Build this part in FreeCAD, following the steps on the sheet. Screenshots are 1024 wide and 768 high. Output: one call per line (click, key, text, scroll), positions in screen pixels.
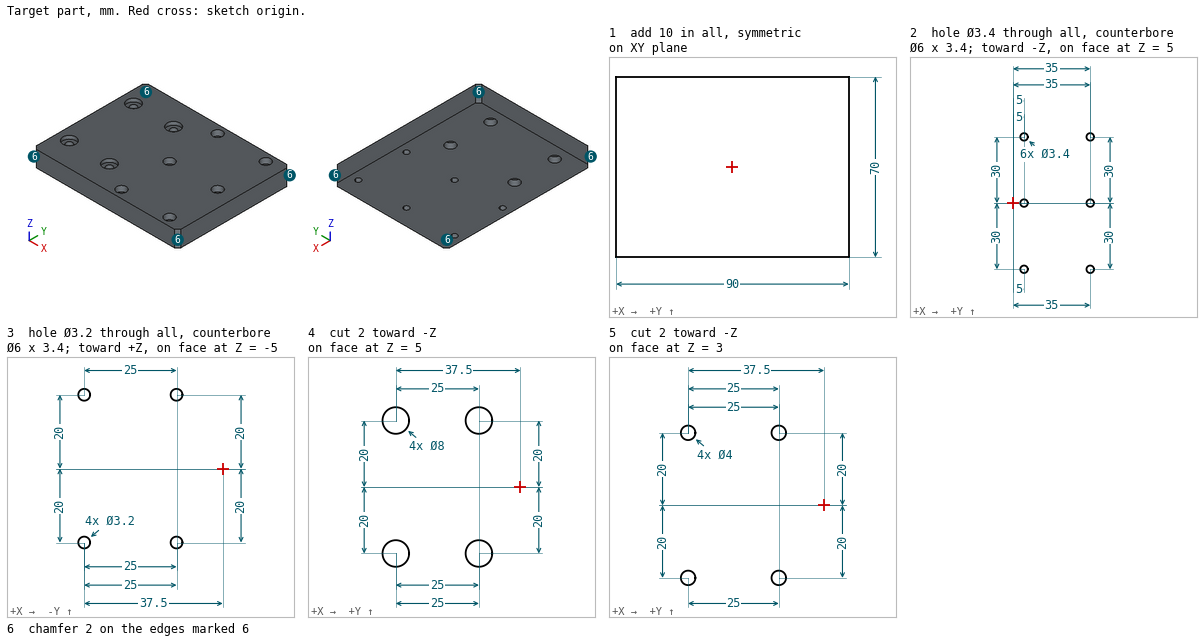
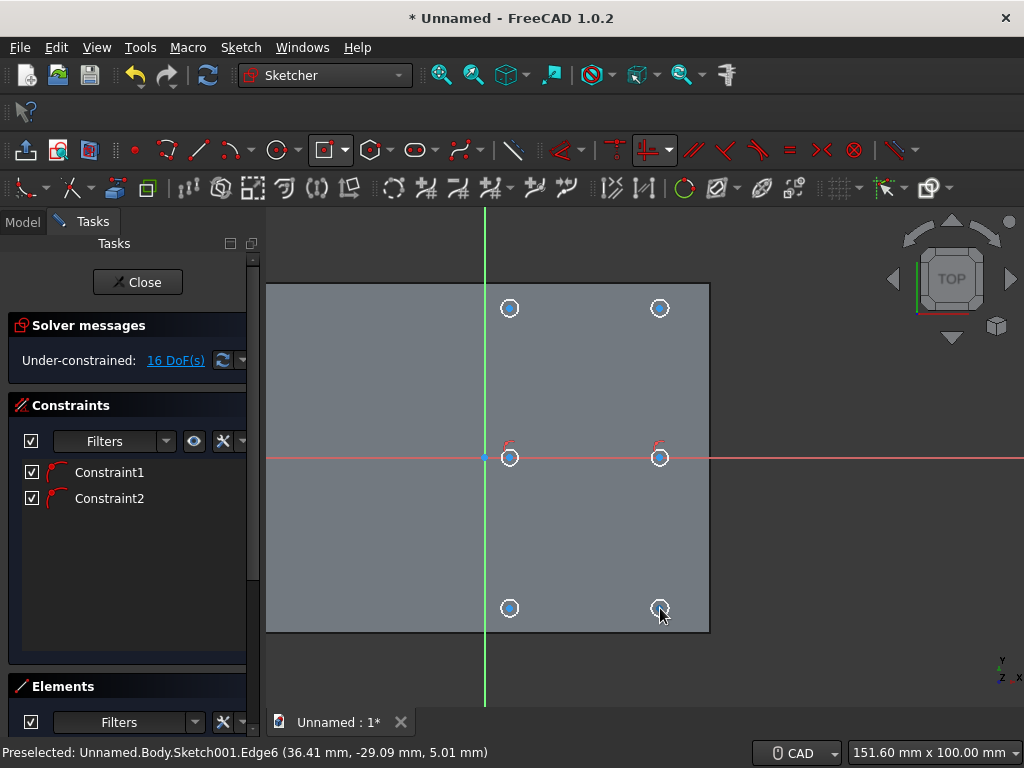
scroll(516, 302, up, 3)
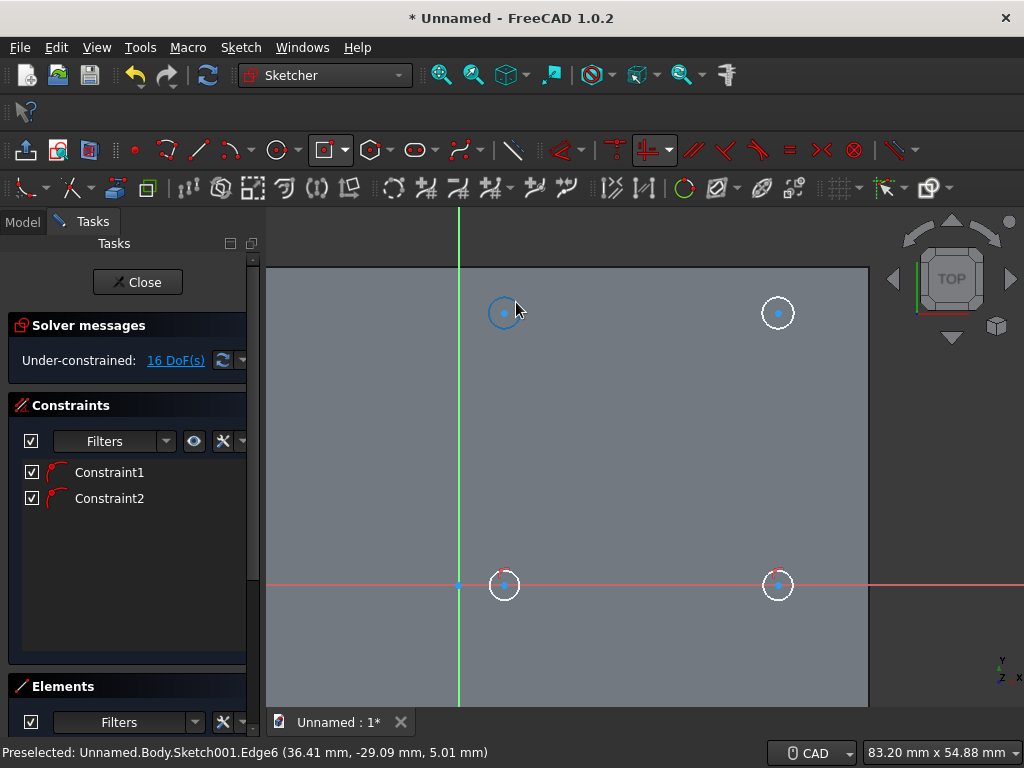
click(516, 302)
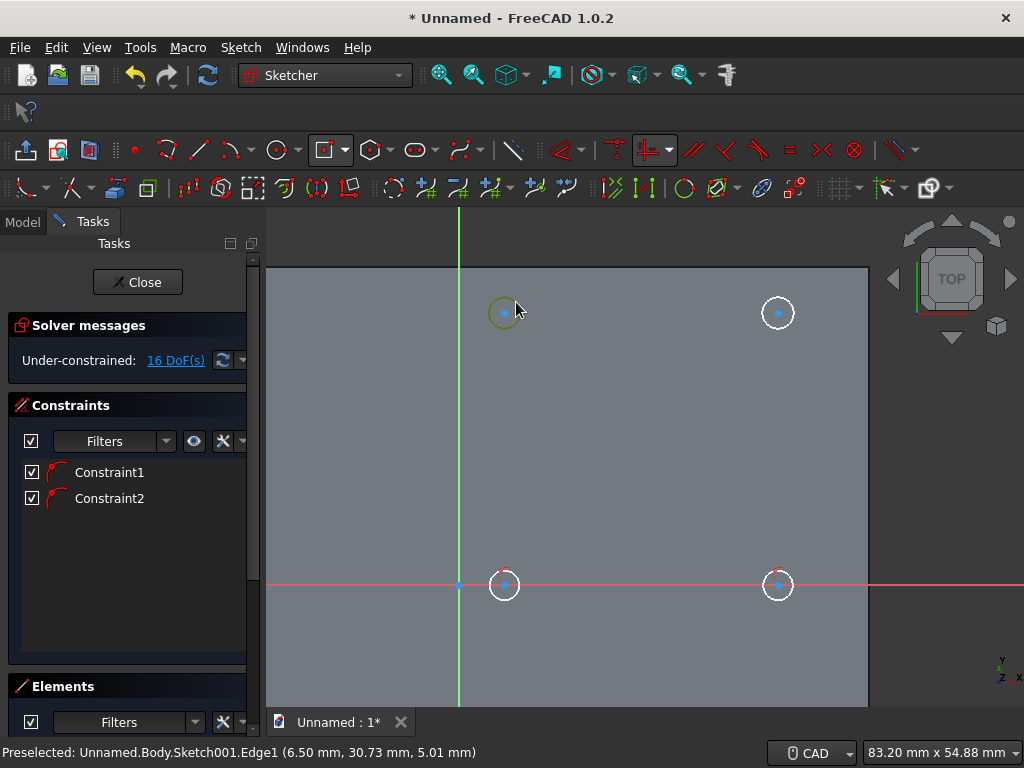
scroll(515, 575, up, 2)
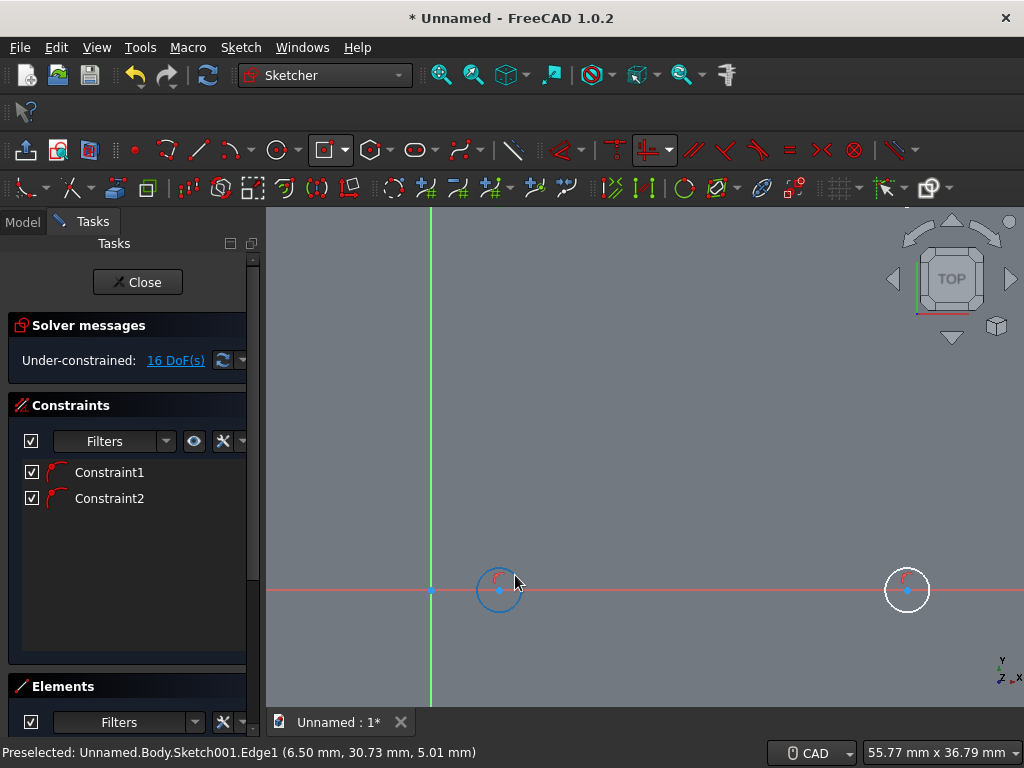
click(515, 575)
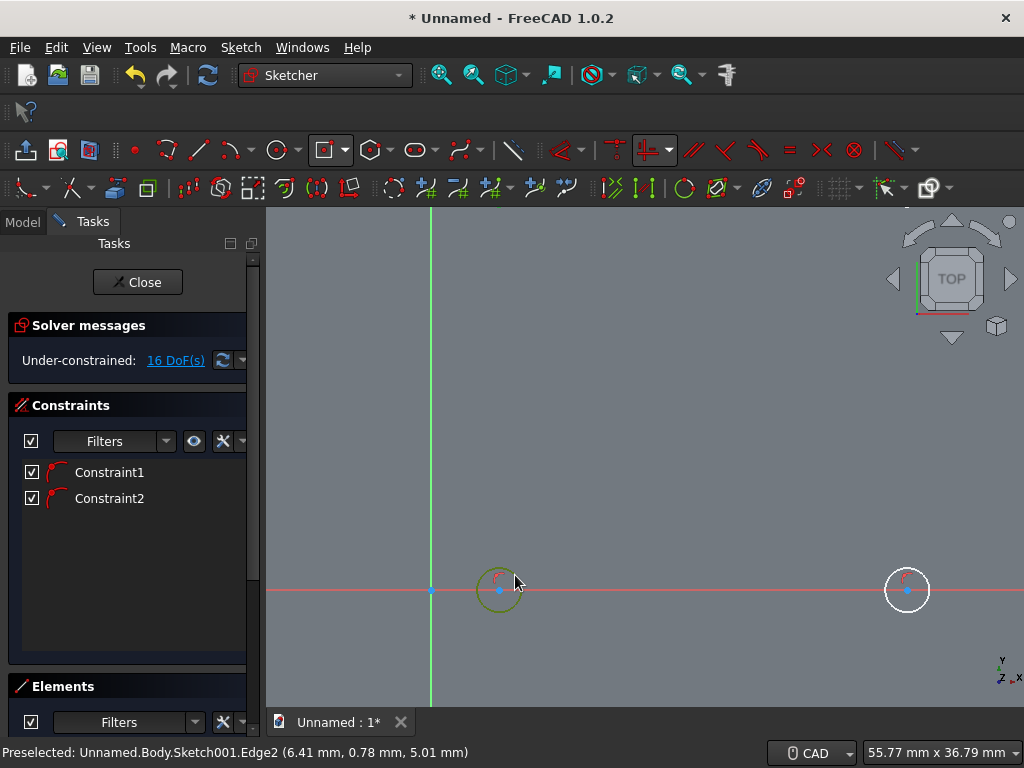
scroll(516, 379, down, 5)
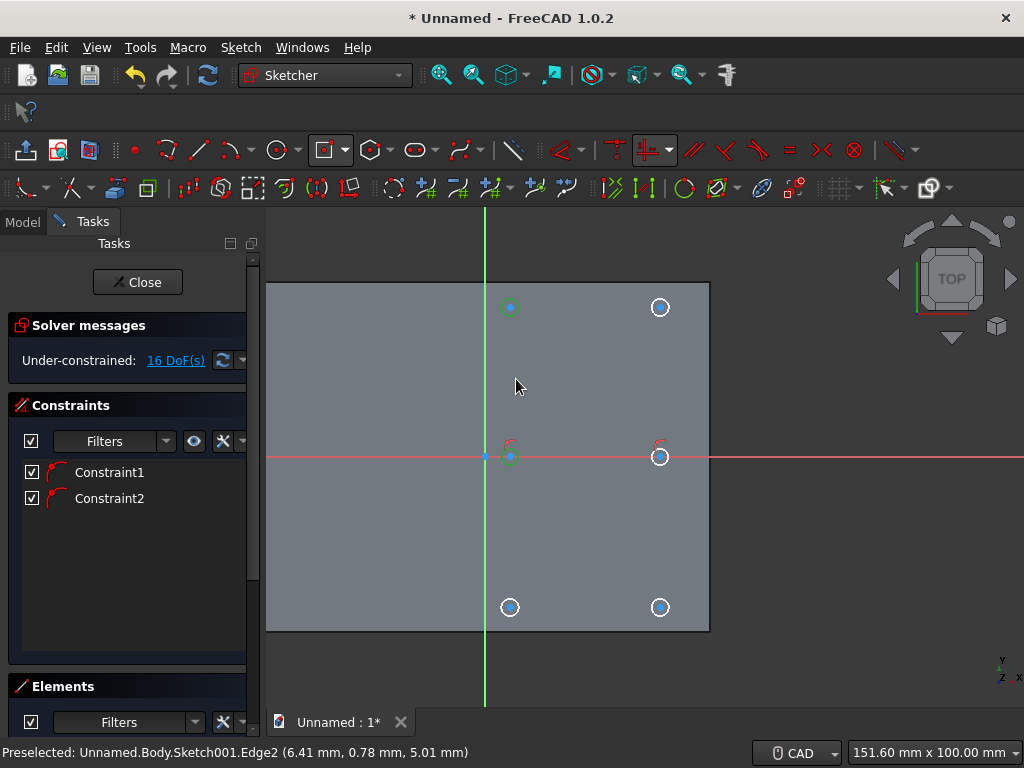
scroll(516, 601, up, 3)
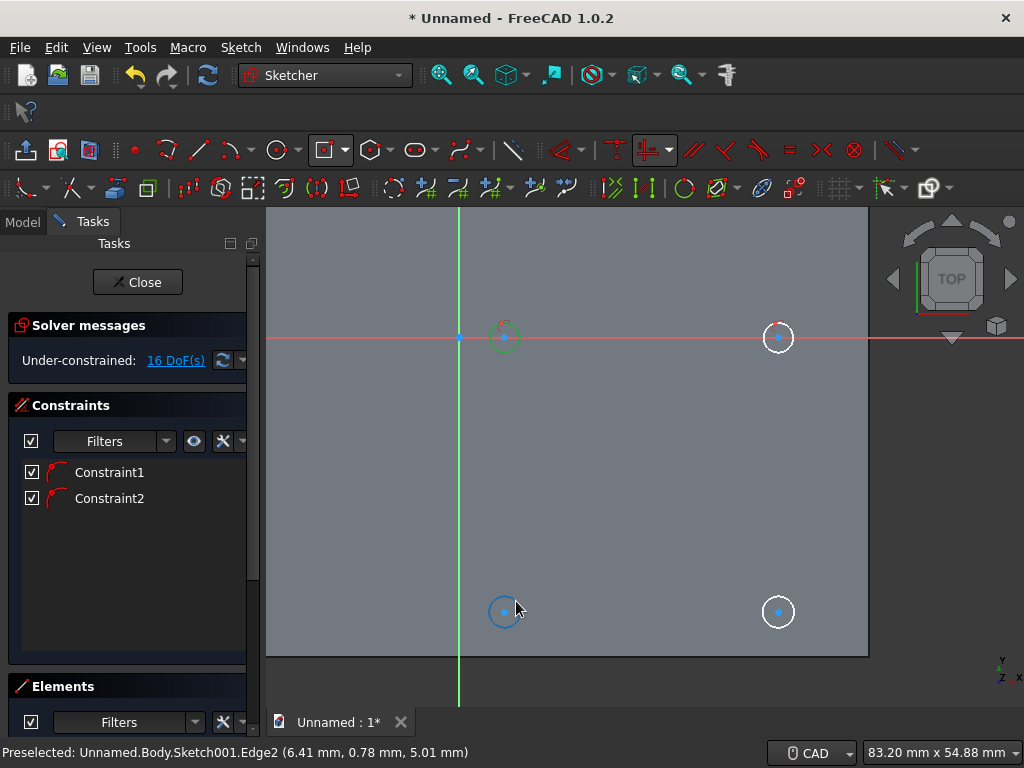
click(516, 601)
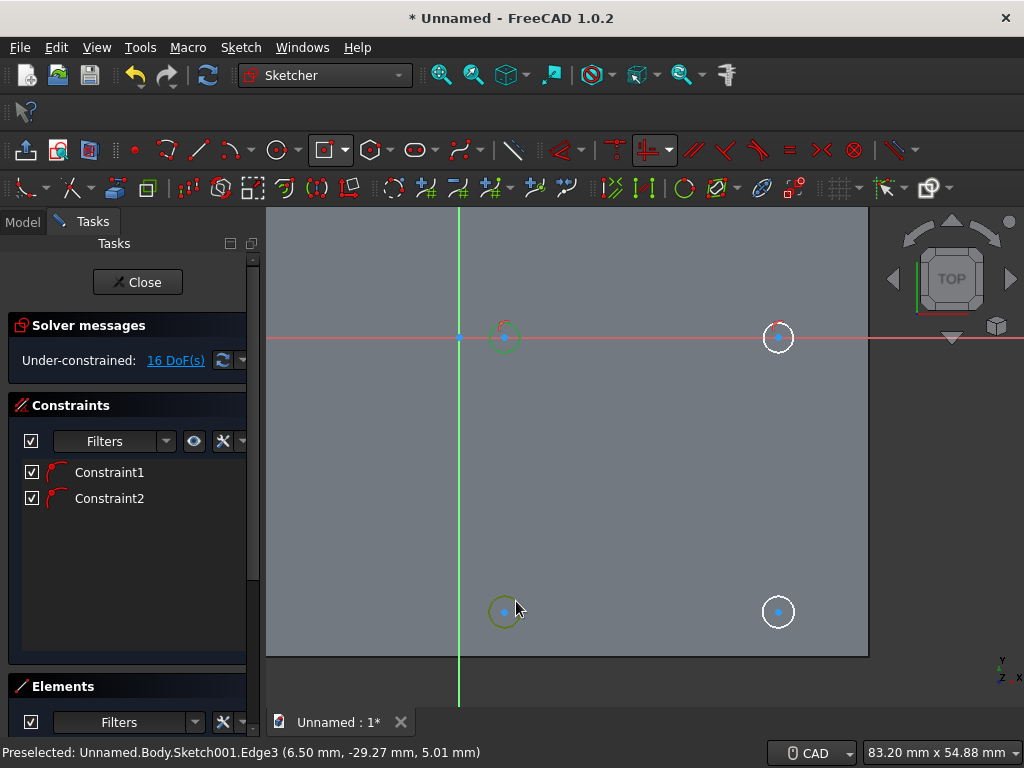
scroll(516, 602, down, 3)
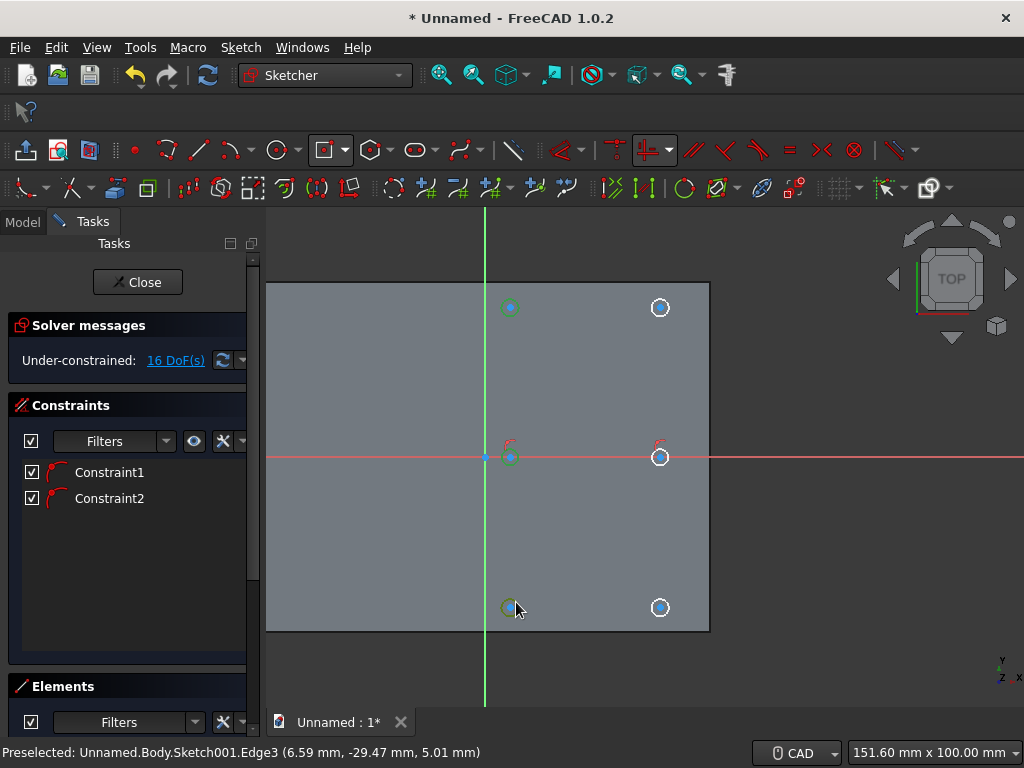
scroll(666, 302, up, 3)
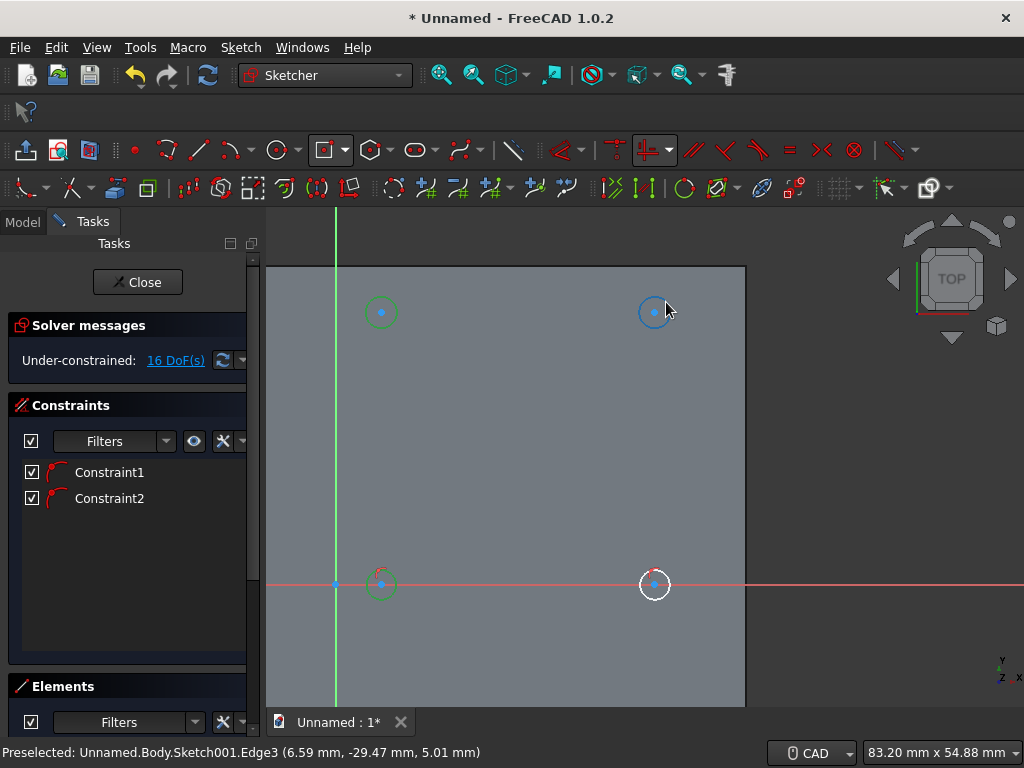
click(666, 301)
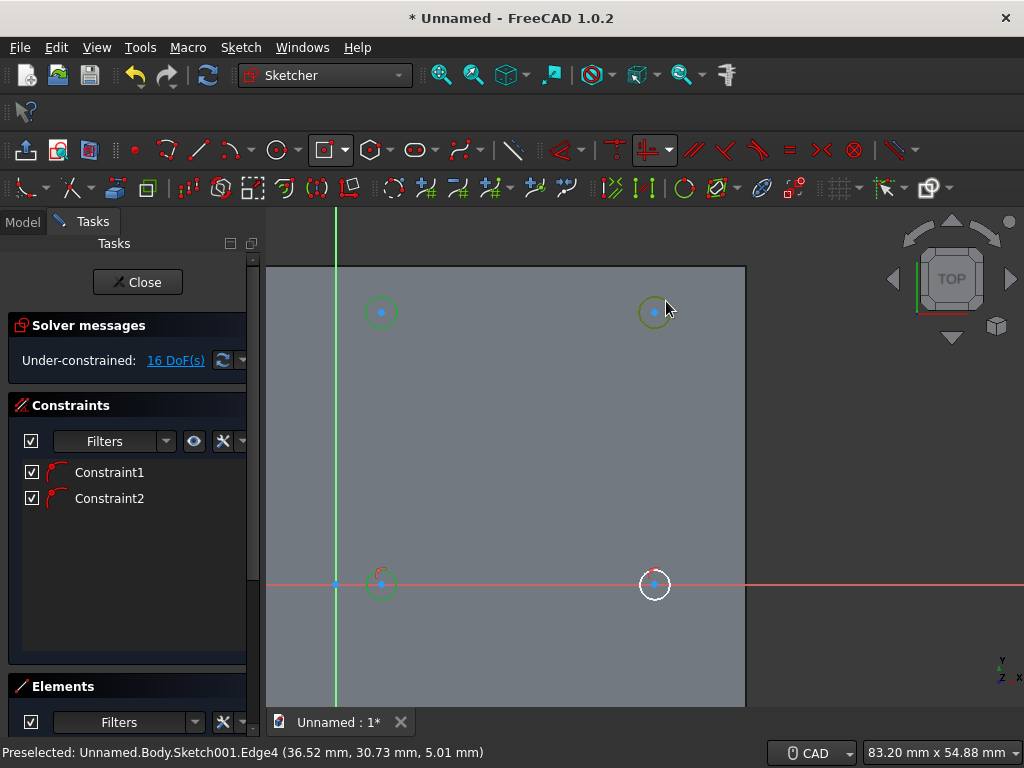
scroll(665, 574, up, 2)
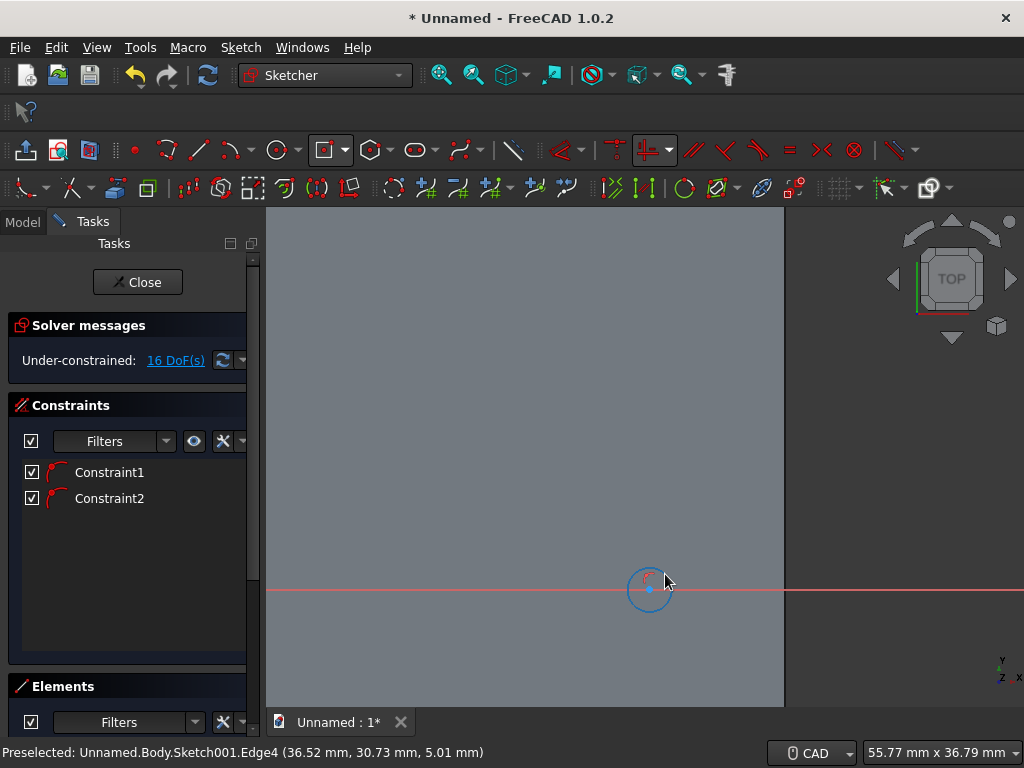
click(665, 574)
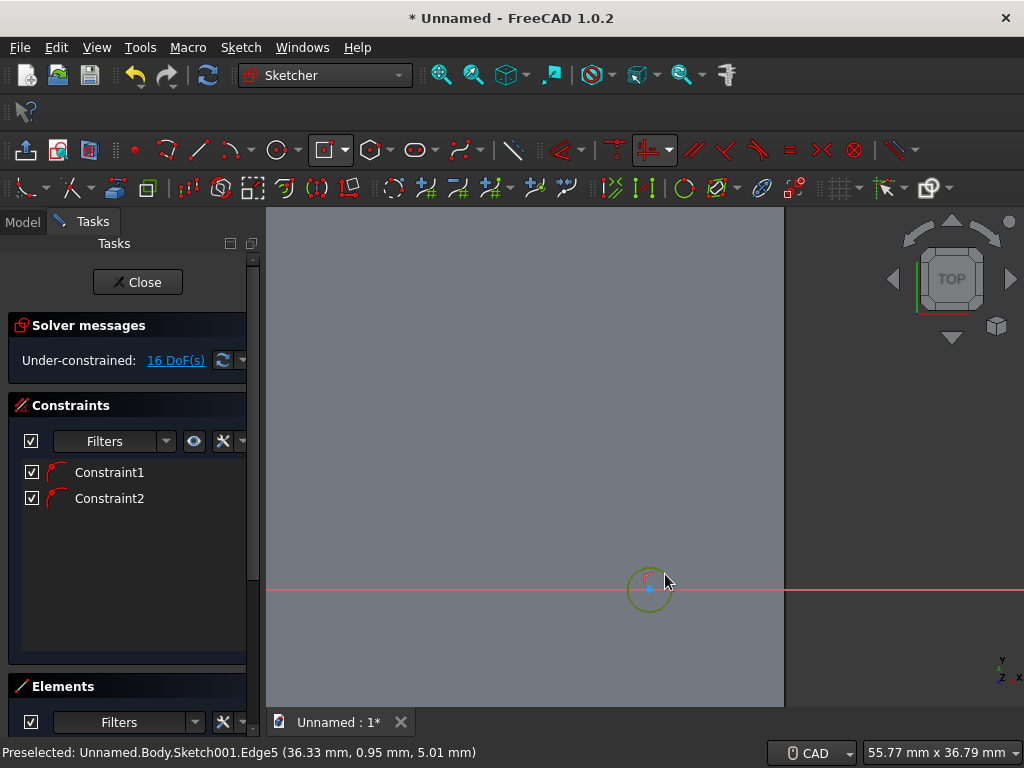
scroll(666, 380, down, 5)